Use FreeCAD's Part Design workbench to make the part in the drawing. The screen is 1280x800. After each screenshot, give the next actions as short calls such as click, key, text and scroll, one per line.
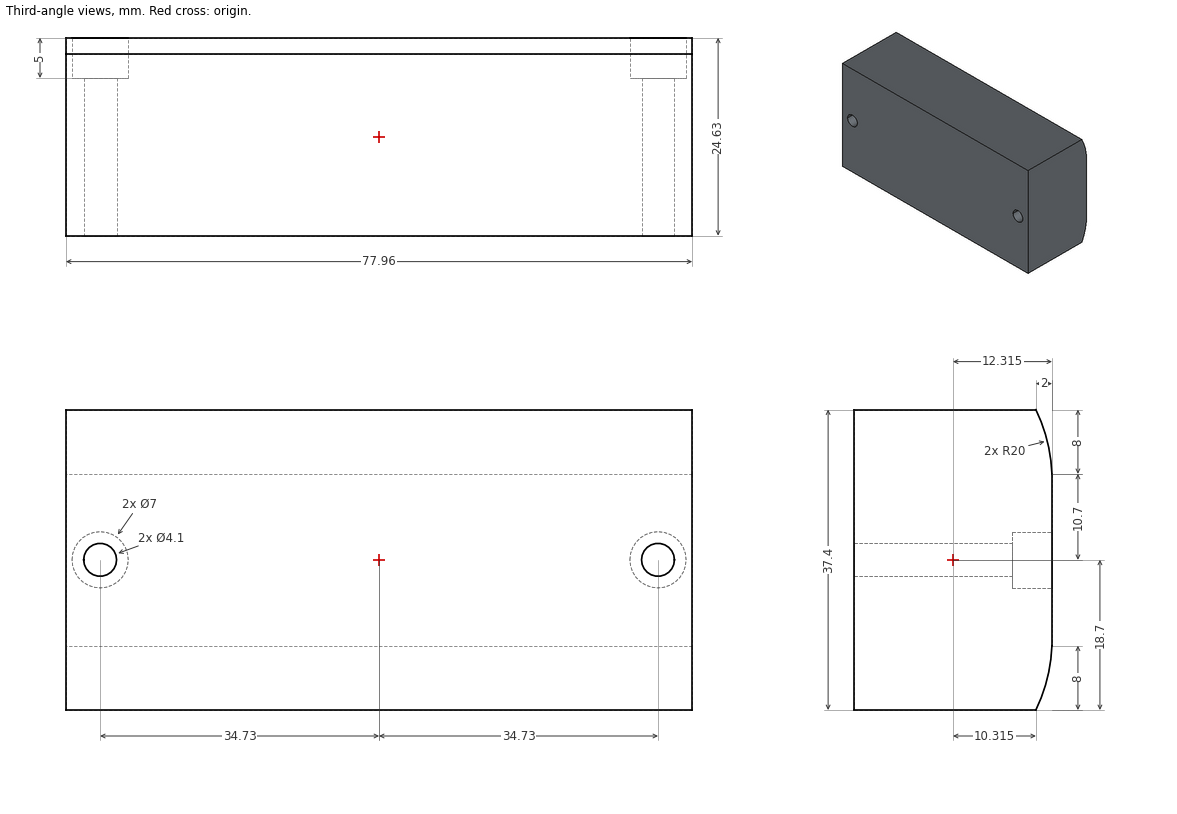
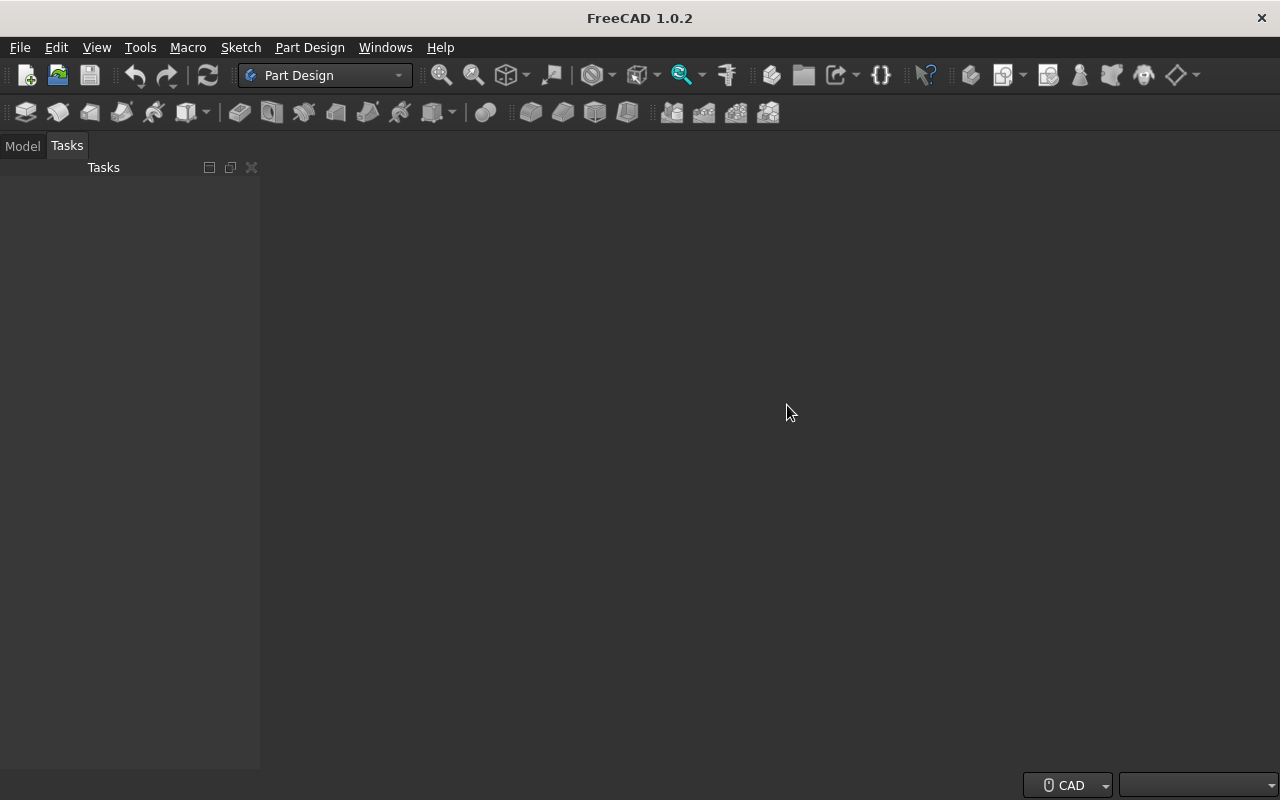
click(26, 76)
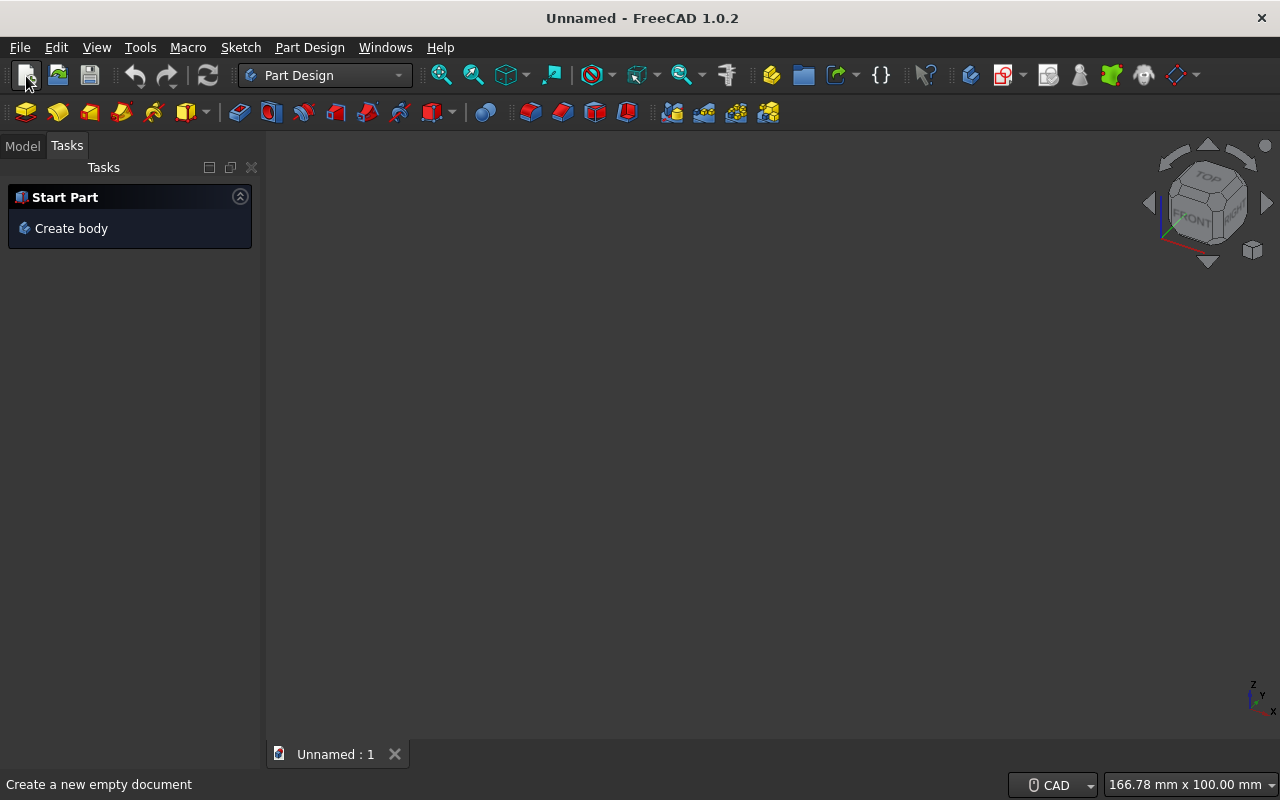
click(1004, 76)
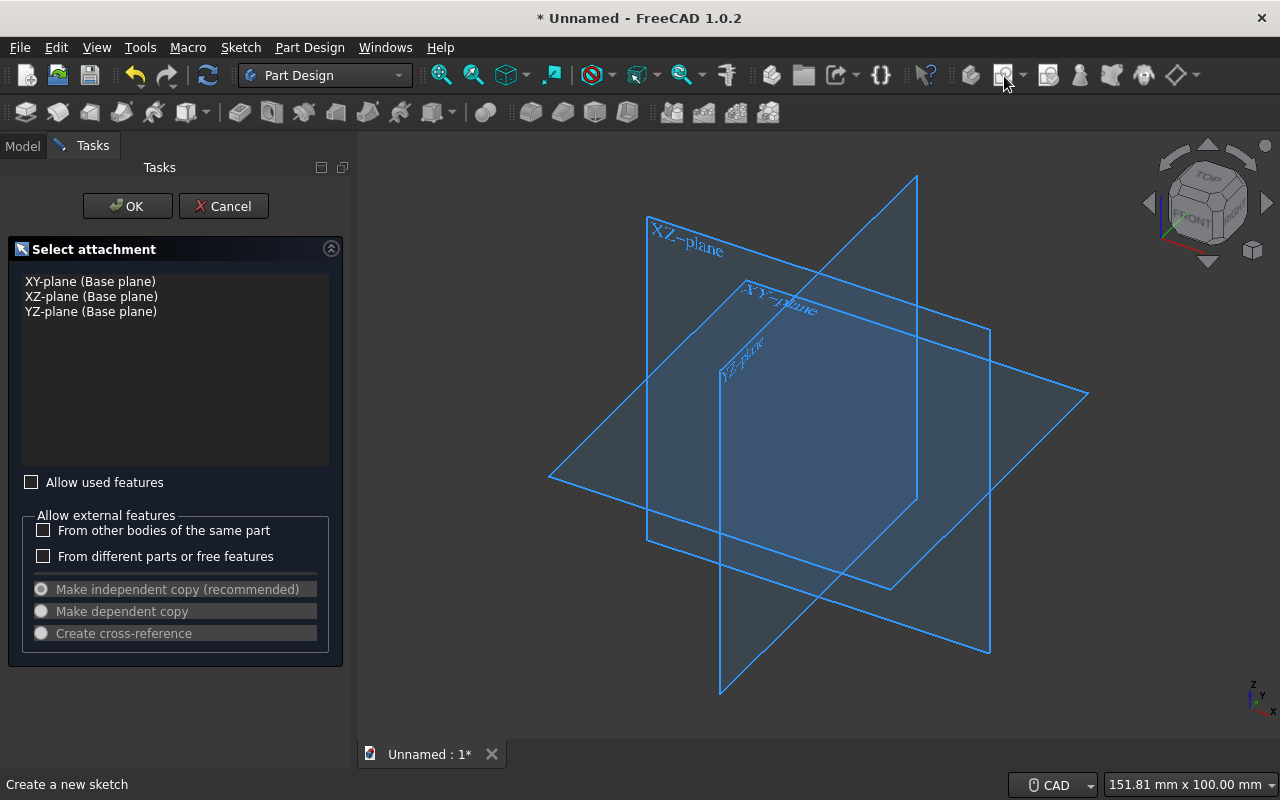
click(82, 282)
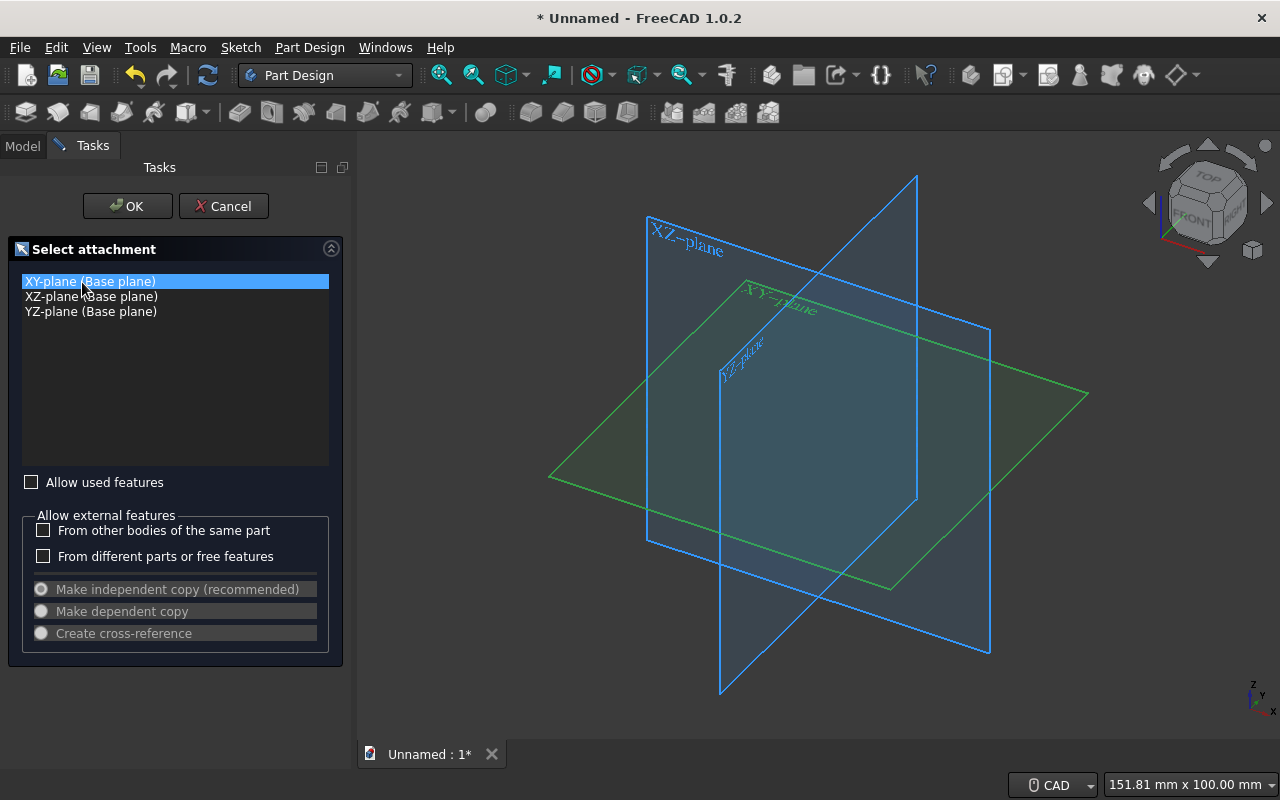
click(128, 206)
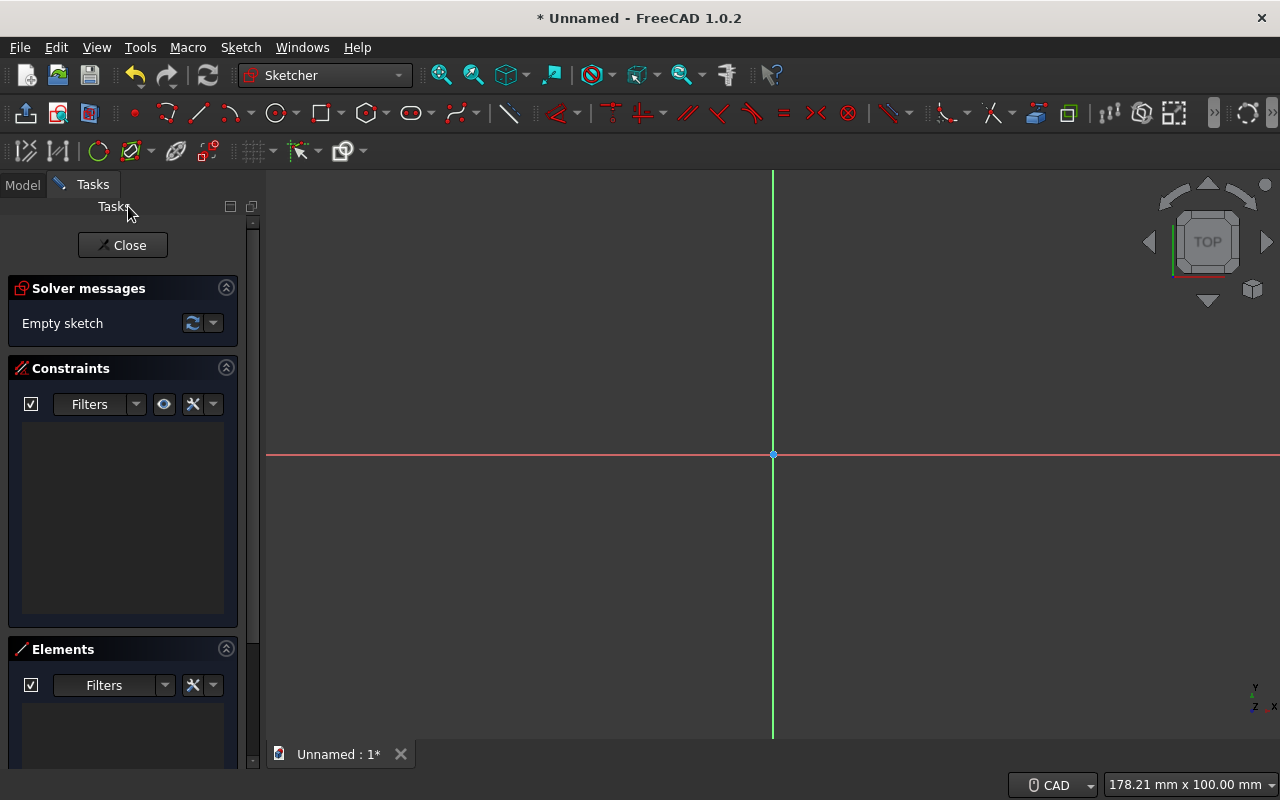
key(g)
key(v)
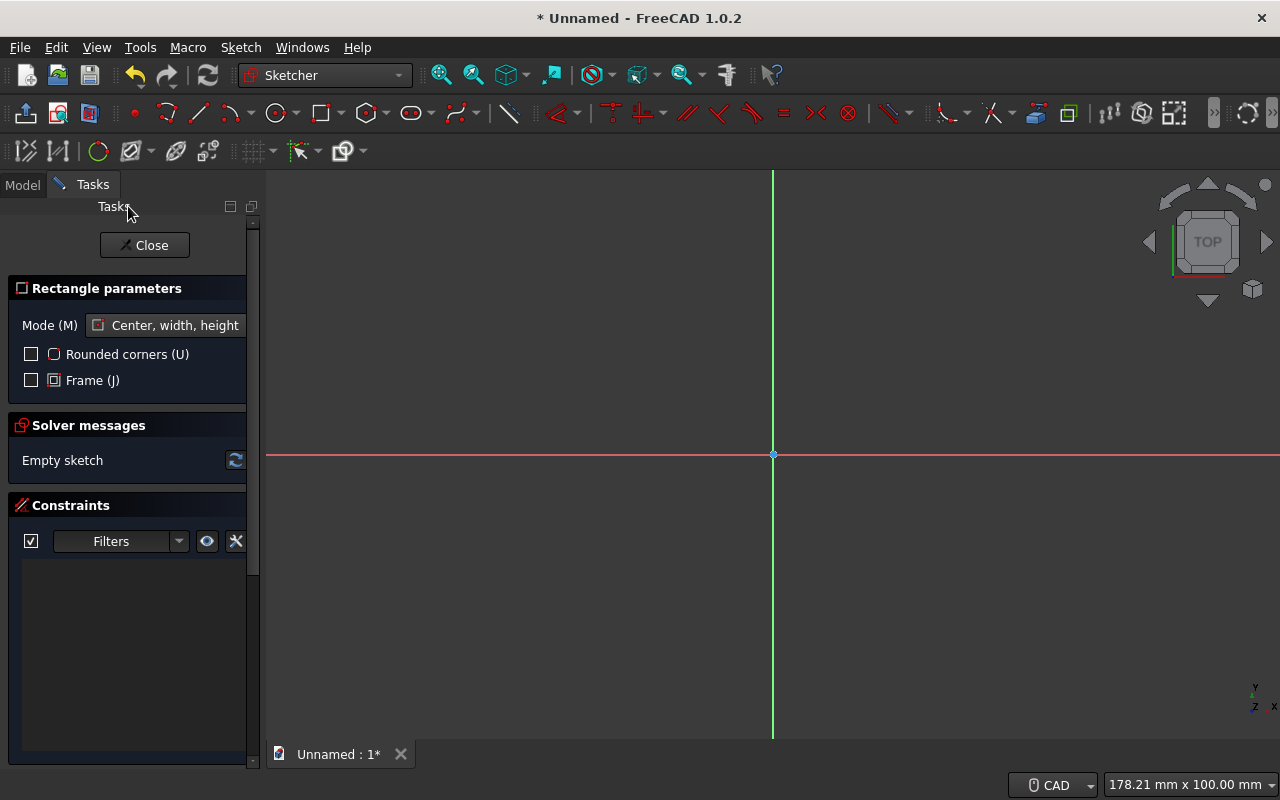
click(773, 454)
click(995, 384)
key(Escape)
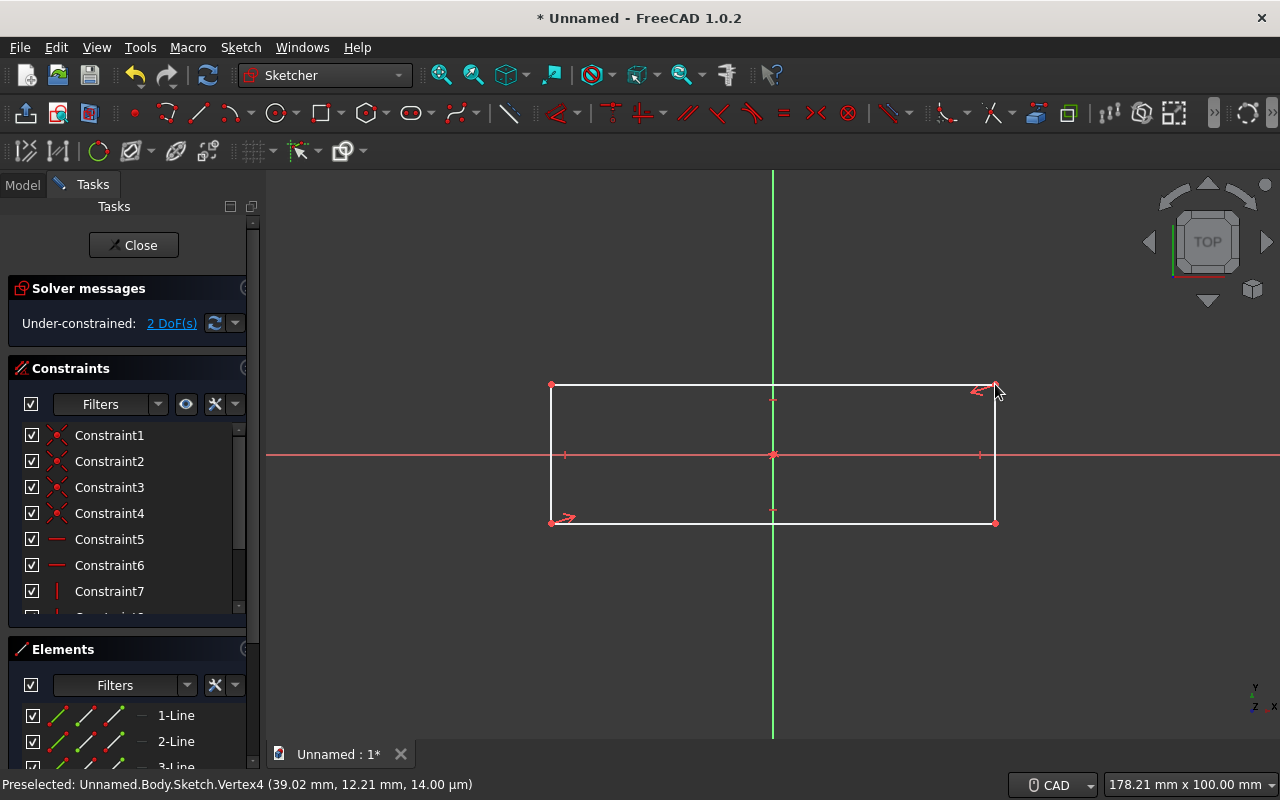
click(684, 524)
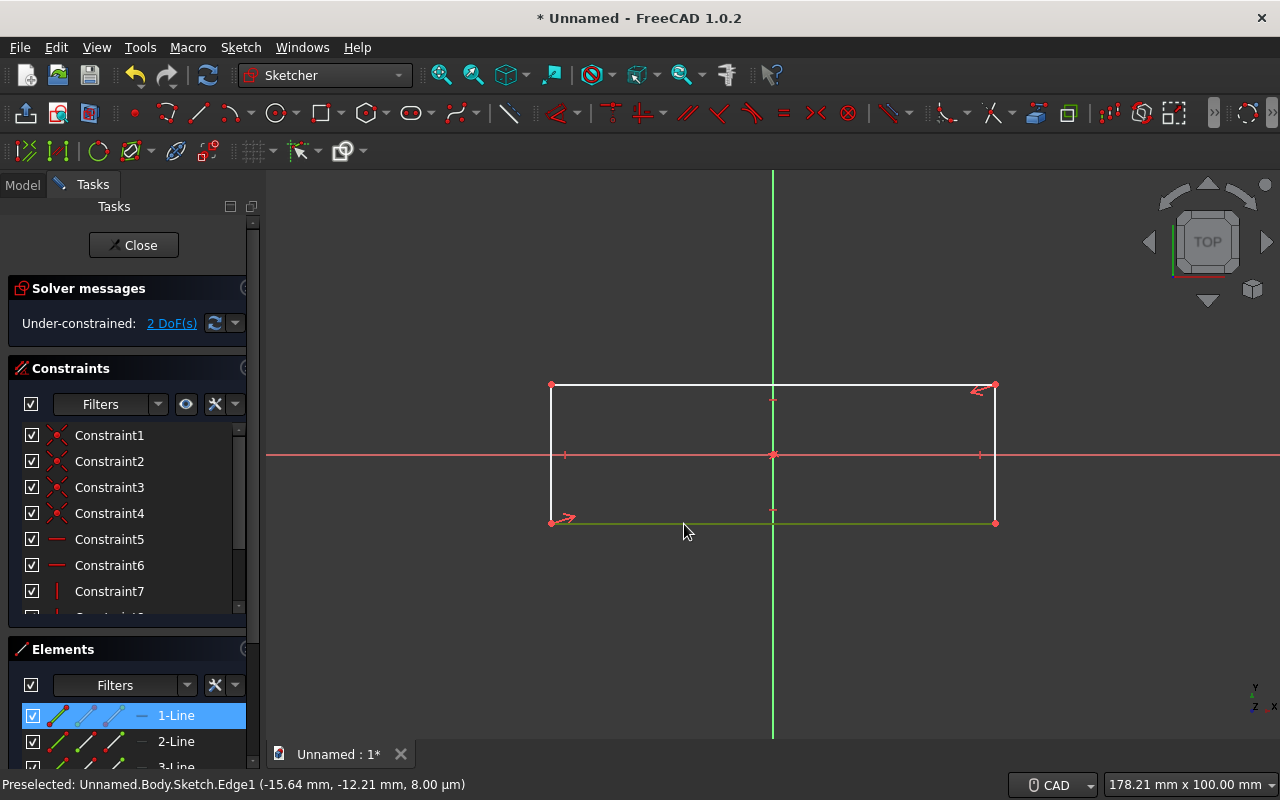
click(580, 114)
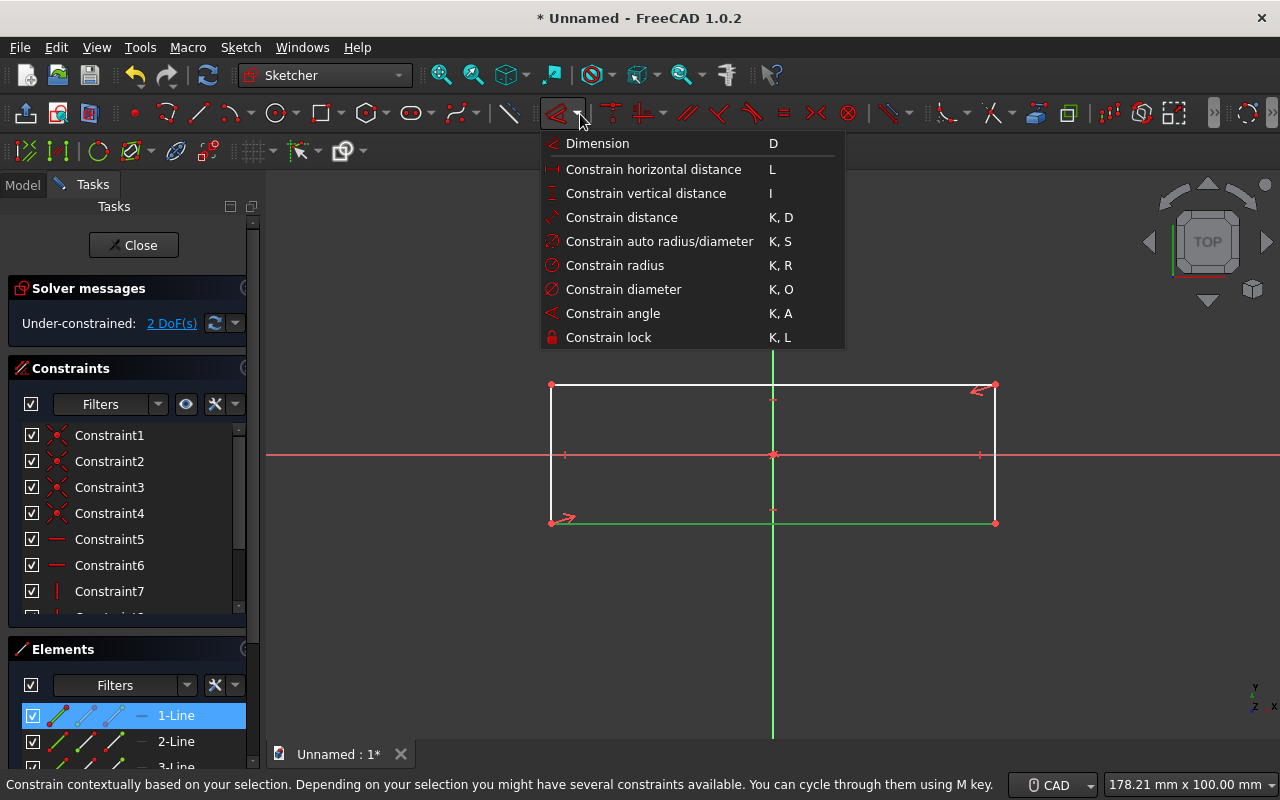
click(693, 169)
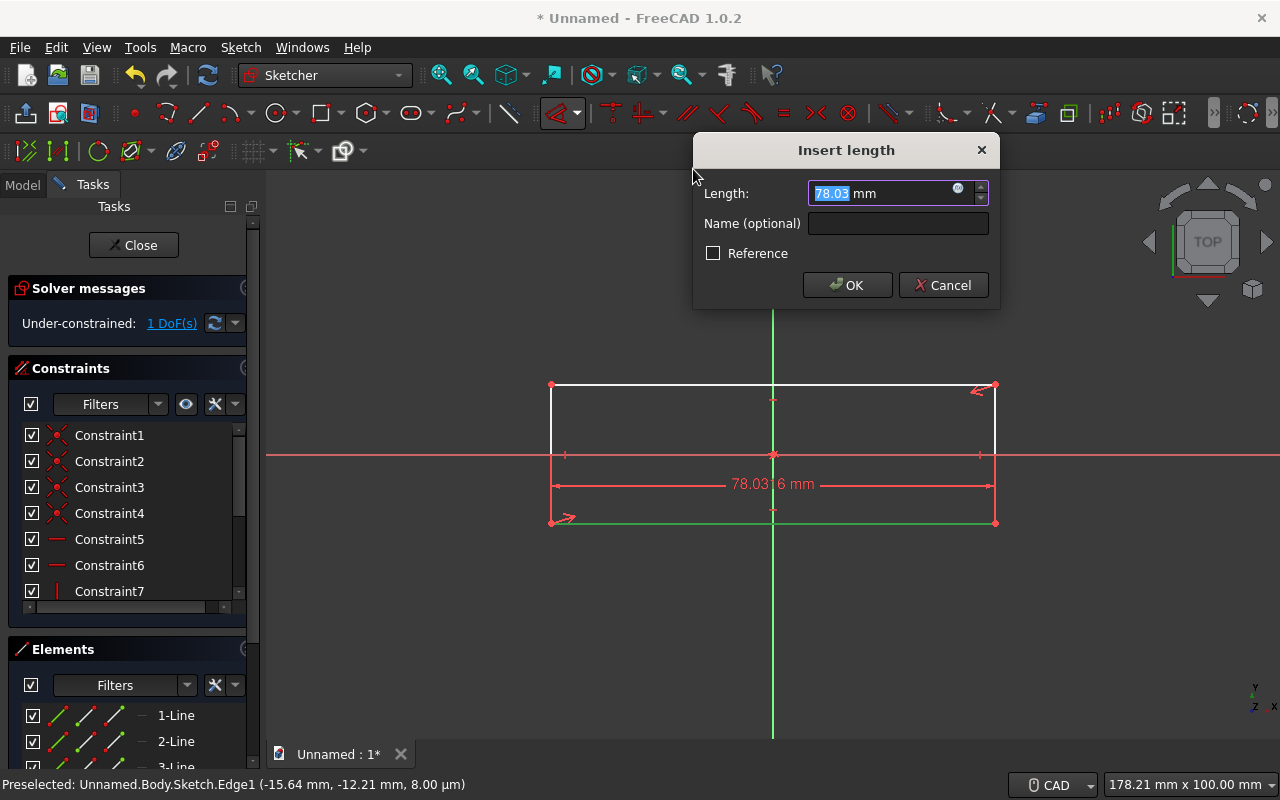
text(77.96)
key(Return)